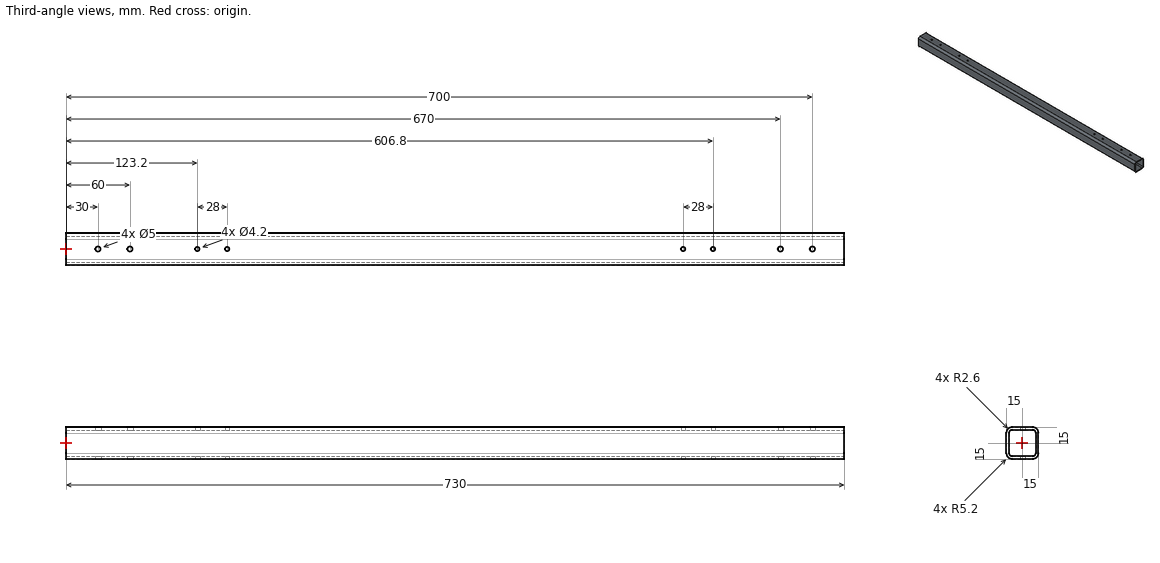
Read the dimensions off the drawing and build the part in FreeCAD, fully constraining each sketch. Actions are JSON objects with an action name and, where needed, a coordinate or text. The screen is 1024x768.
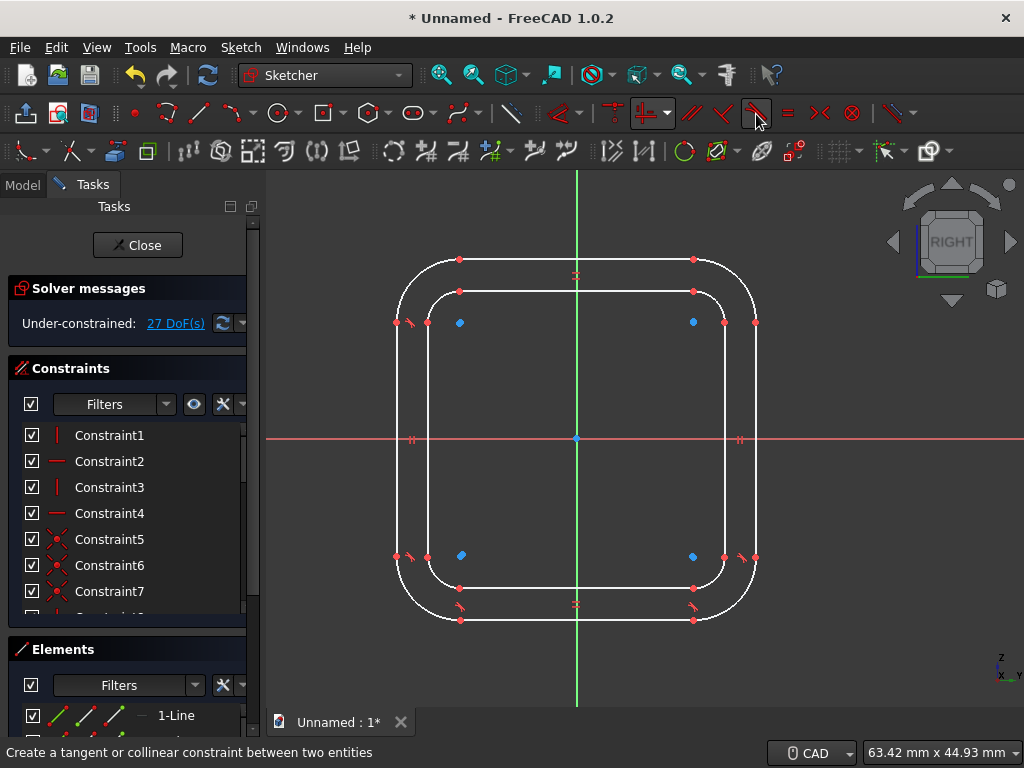
{"action": "left_click", "coordinate": [756, 487]}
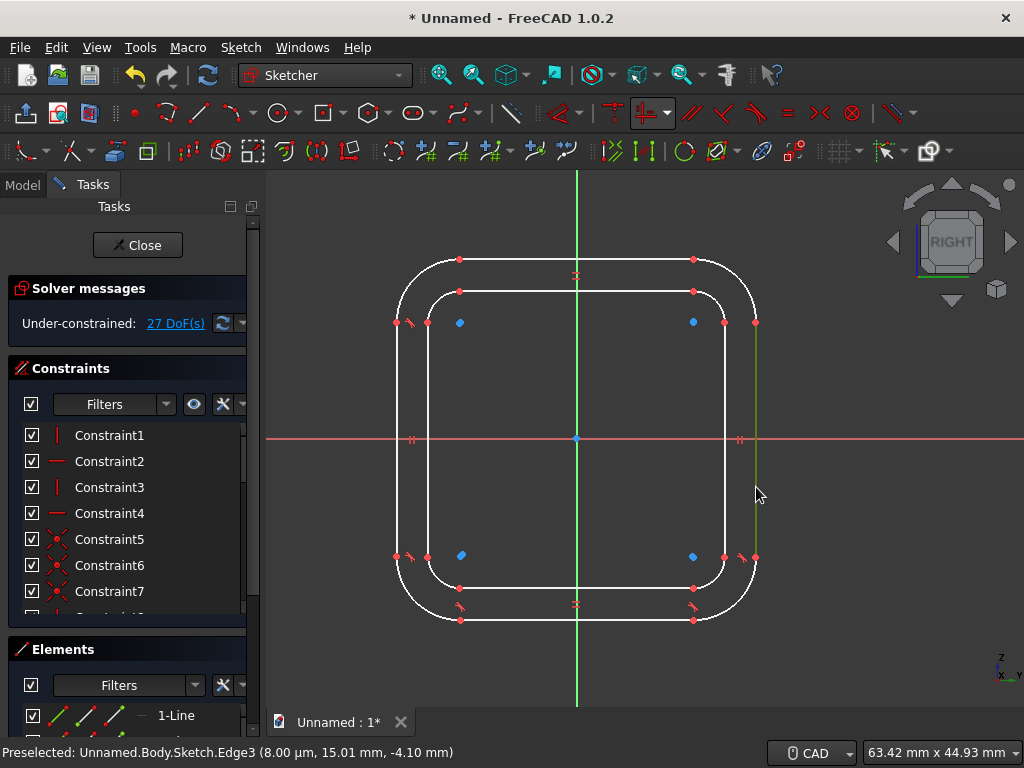
{"action": "left_click", "coordinate": [750, 294]}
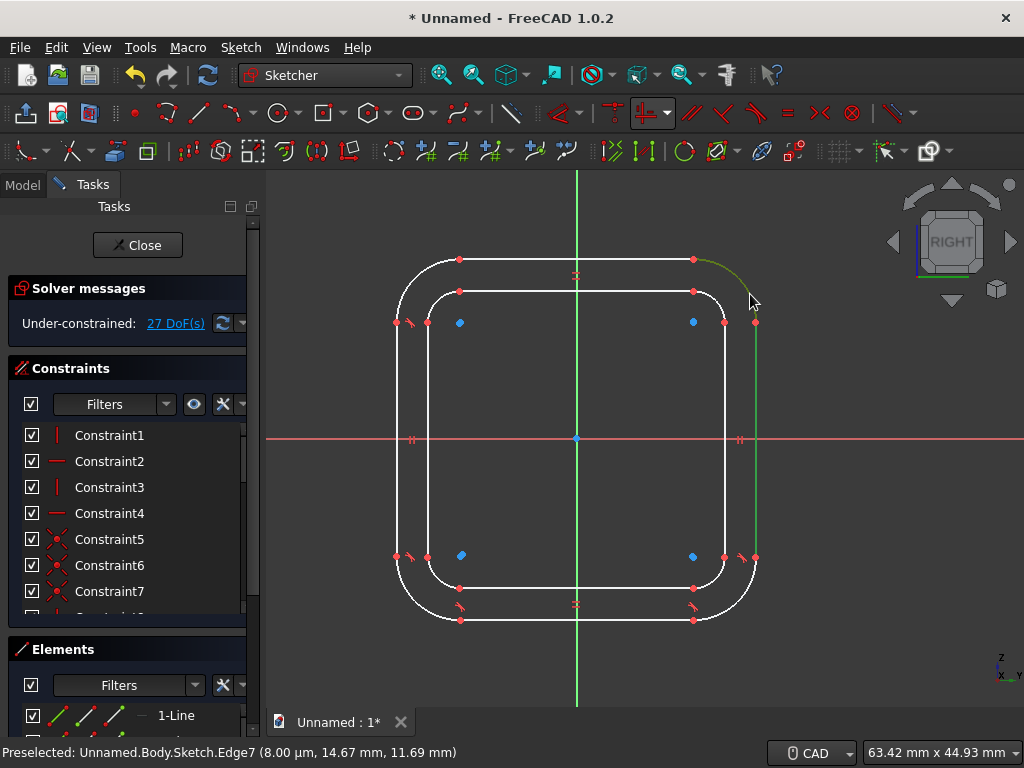
{"action": "left_click", "coordinate": [756, 114]}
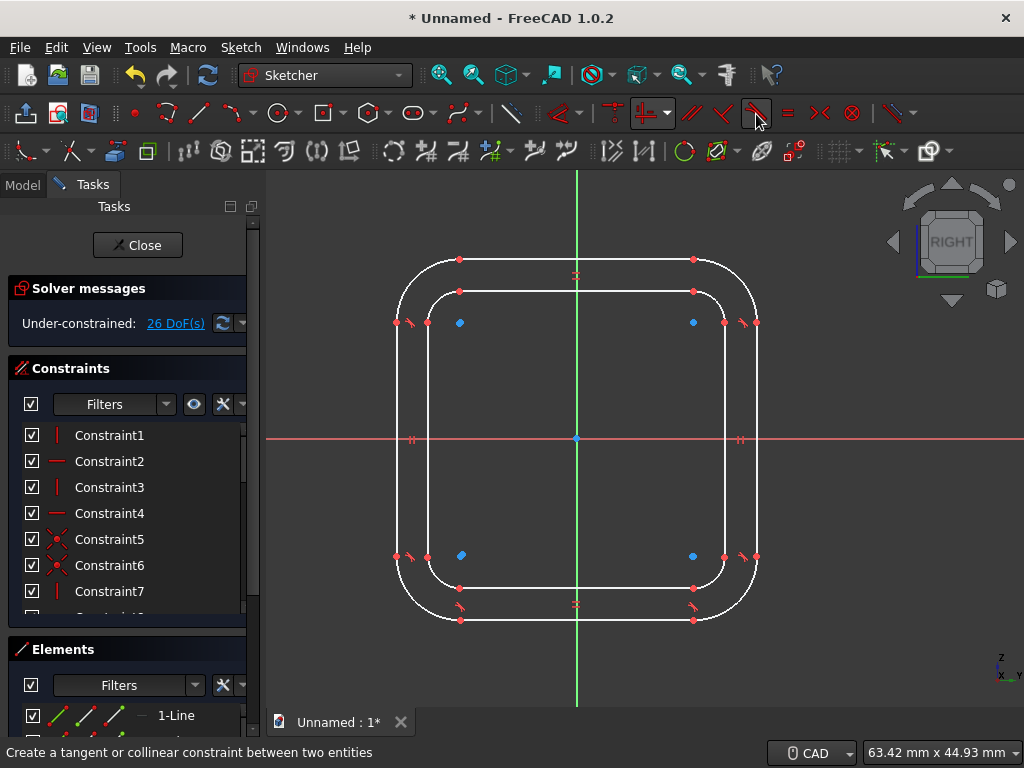
{"action": "left_click", "coordinate": [624, 259]}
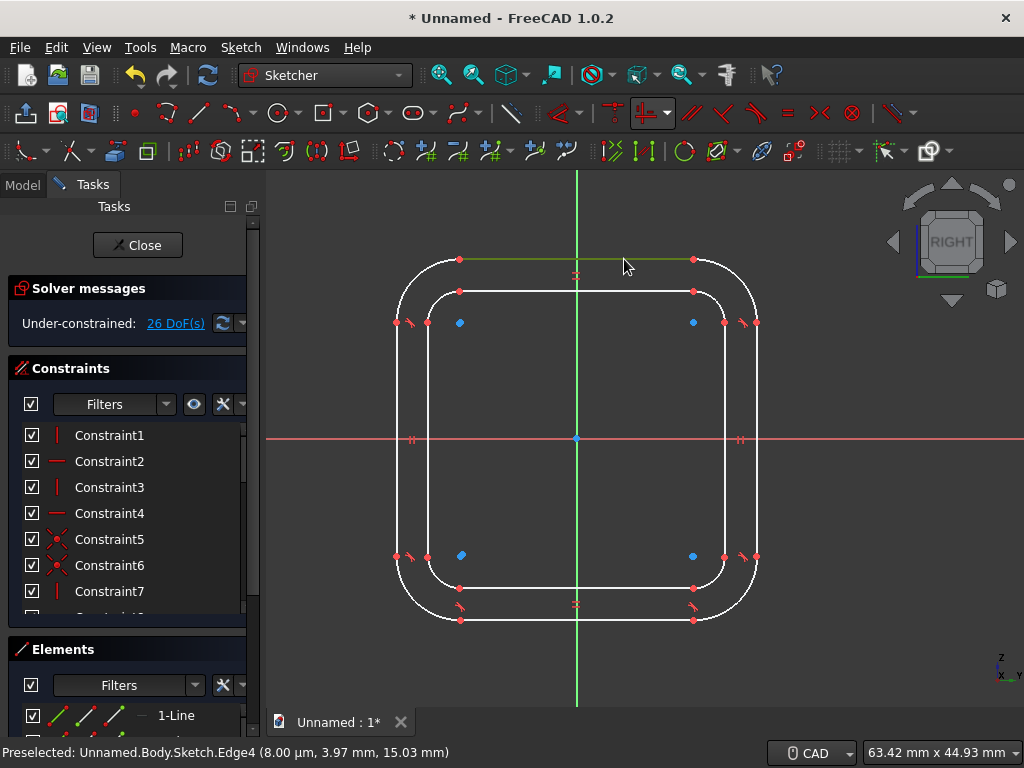
{"action": "left_click", "coordinate": [750, 294]}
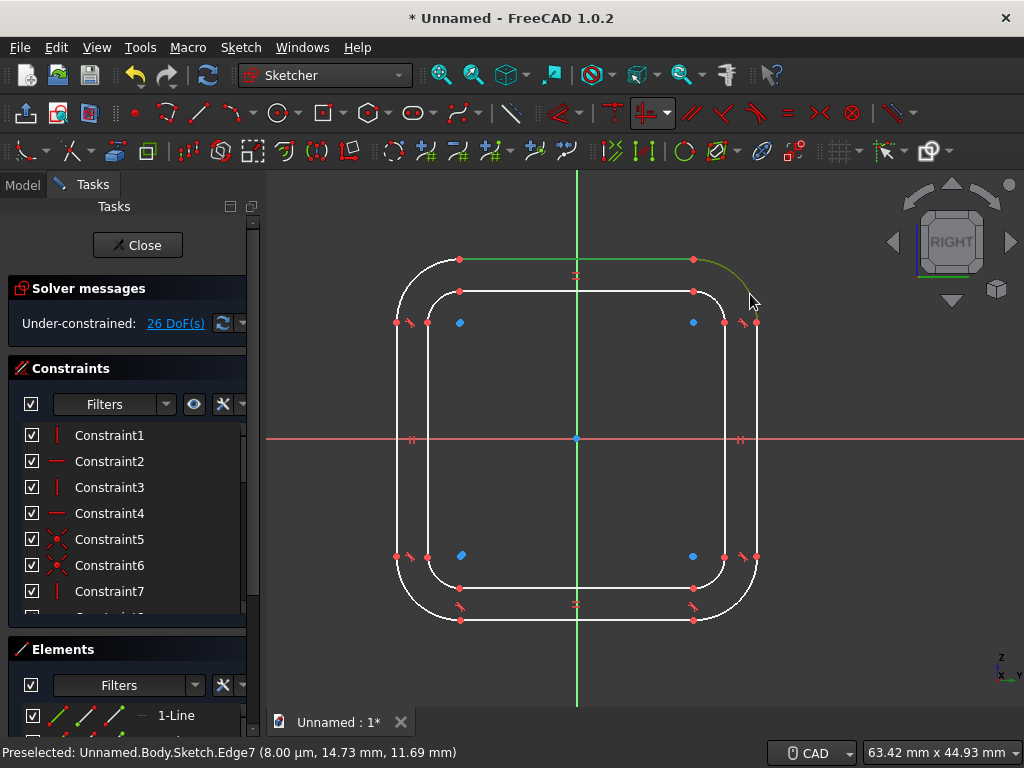
{"action": "left_click", "coordinate": [756, 114]}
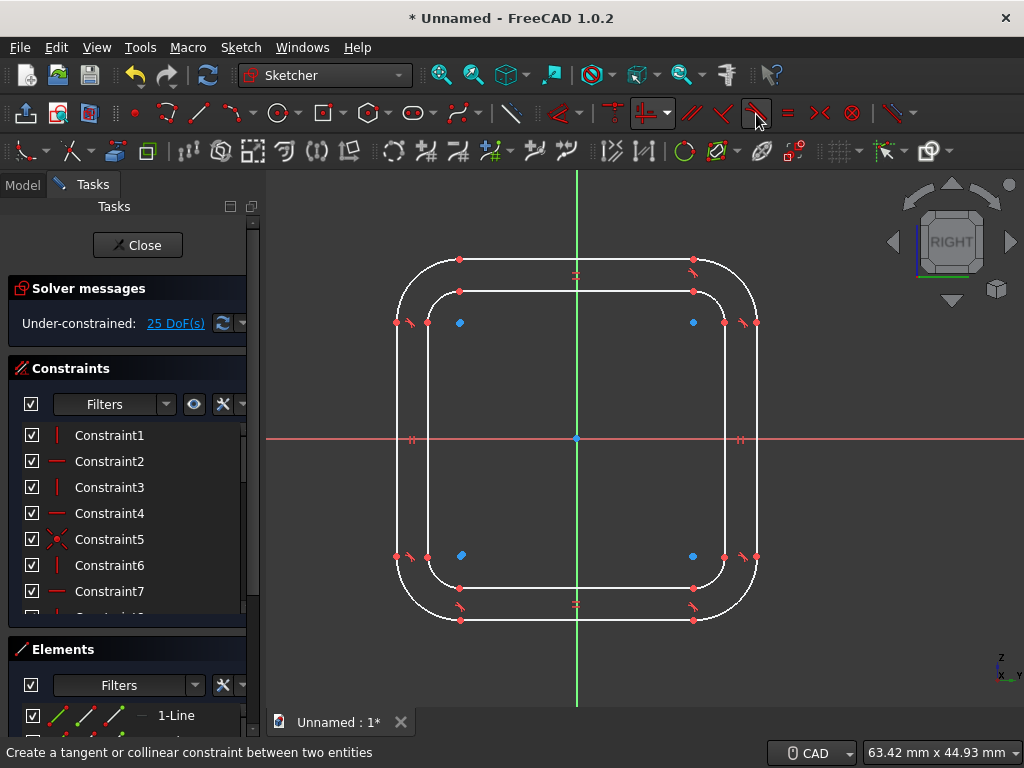
{"action": "left_click", "coordinate": [624, 259]}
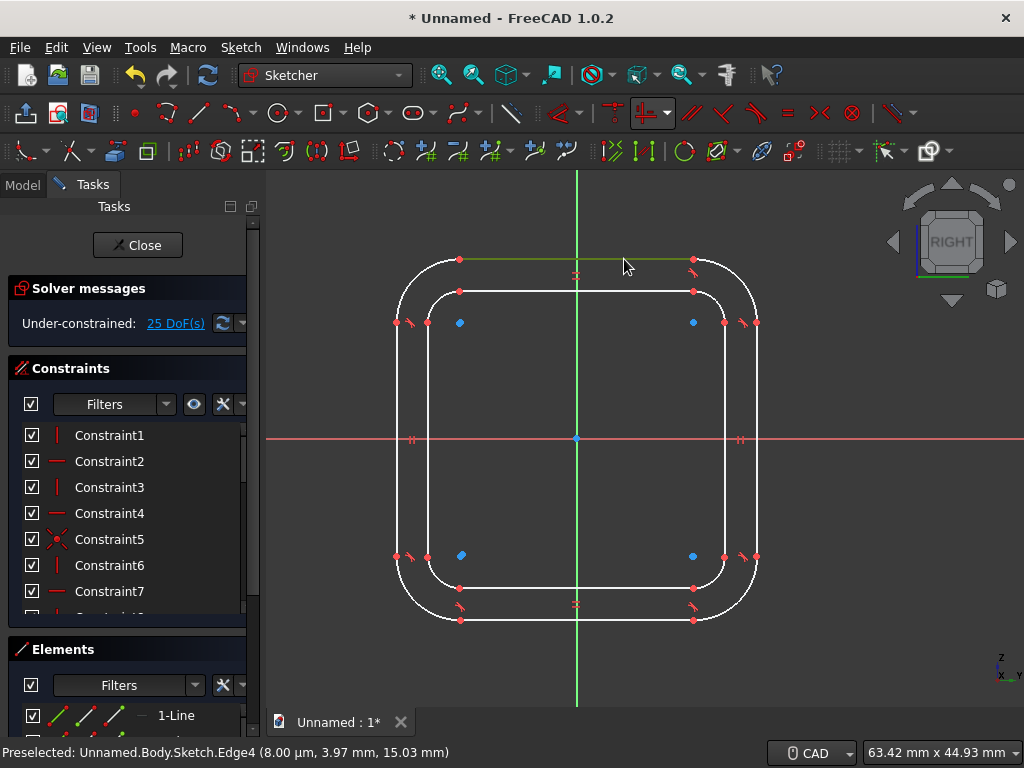
{"action": "left_click", "coordinate": [431, 266]}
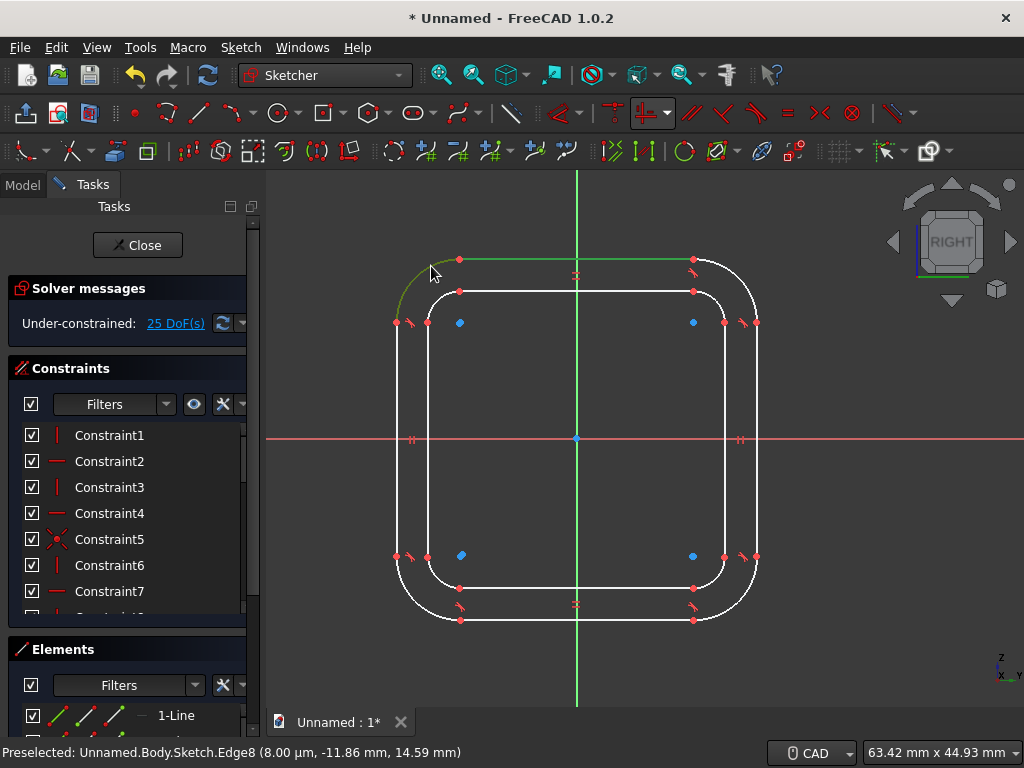
{"action": "left_click", "coordinate": [756, 114]}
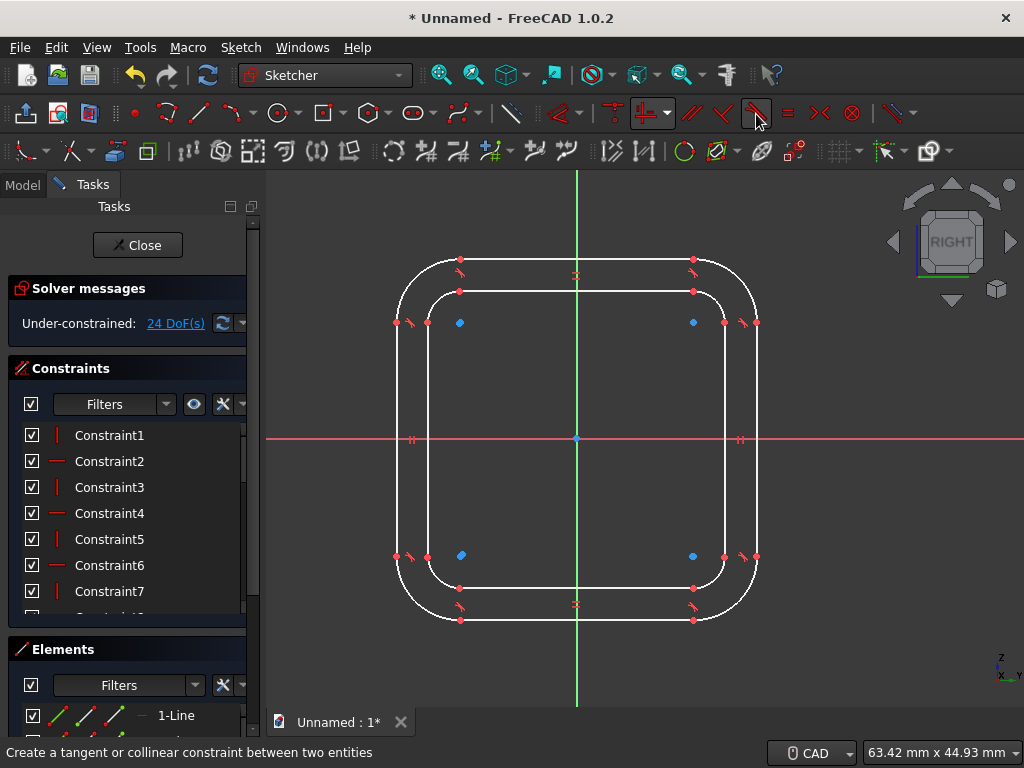
{"action": "left_click", "coordinate": [428, 487]}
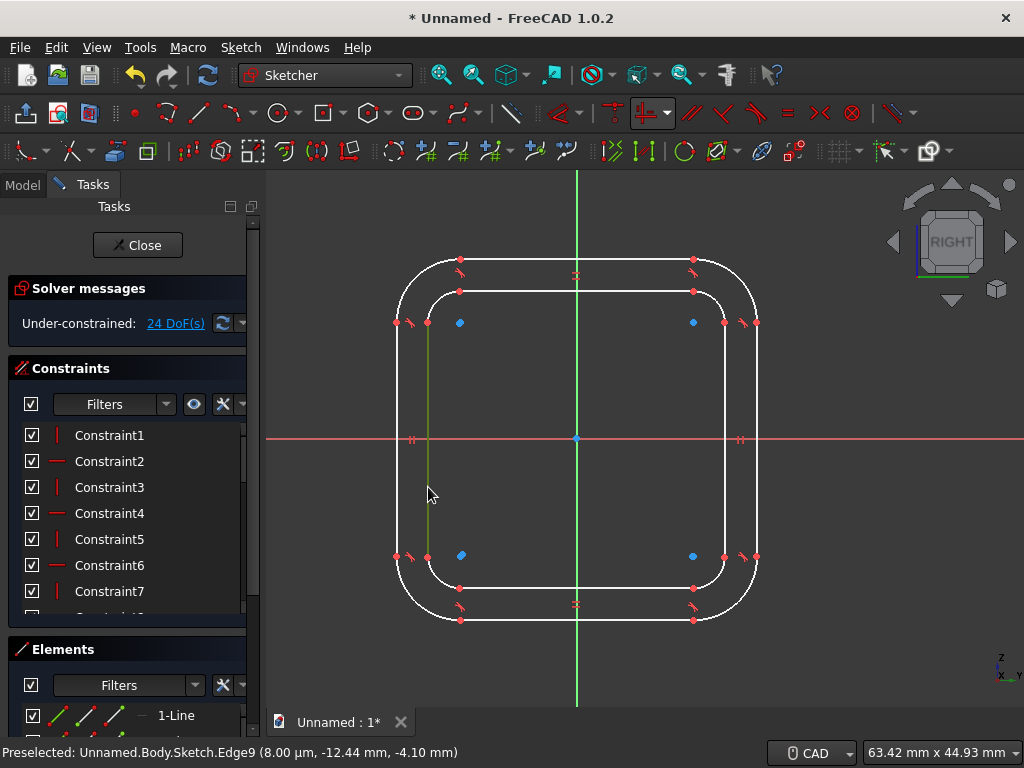
{"action": "left_click", "coordinate": [446, 295]}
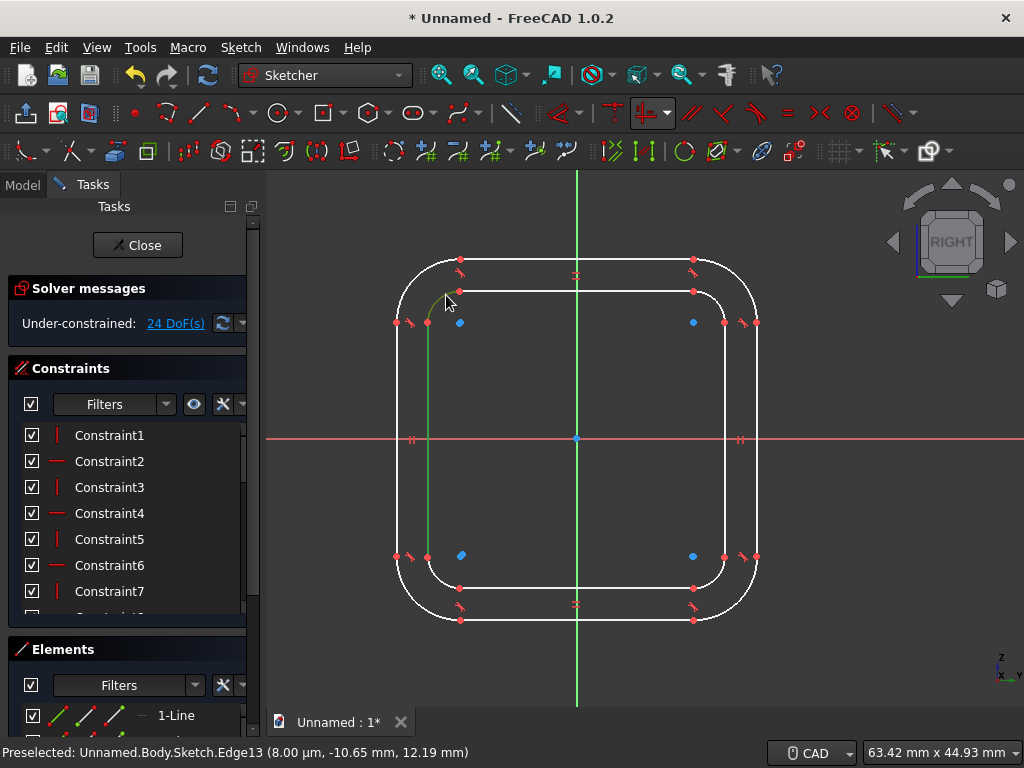
{"action": "left_click", "coordinate": [756, 114]}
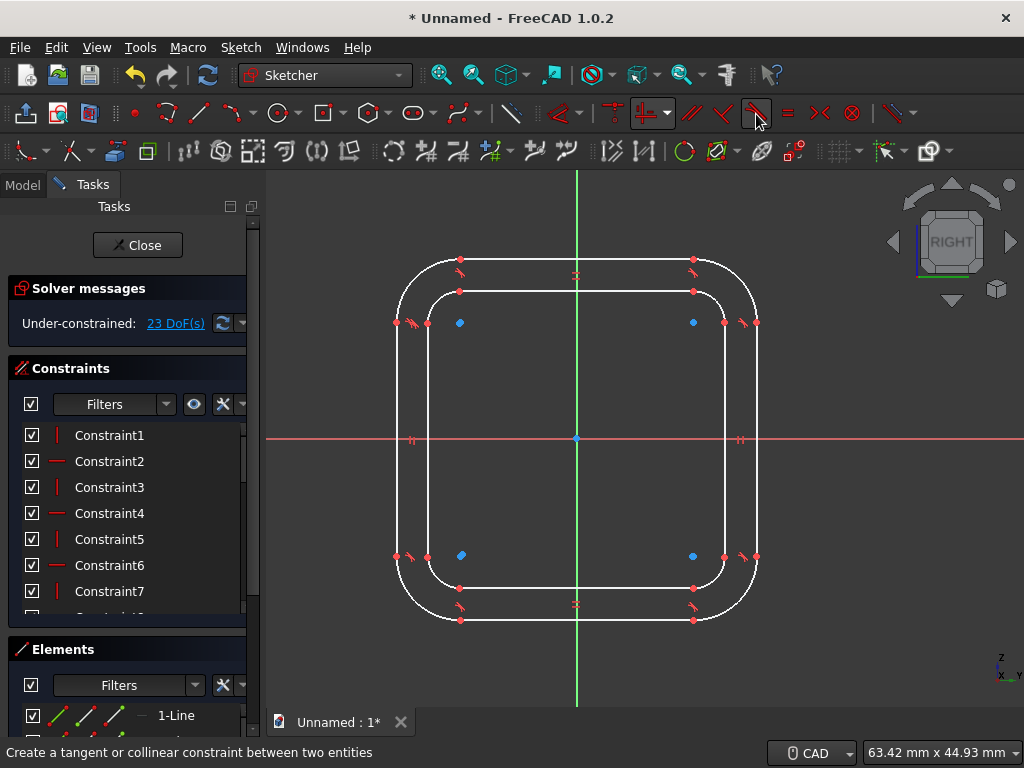
{"action": "left_click", "coordinate": [428, 487]}